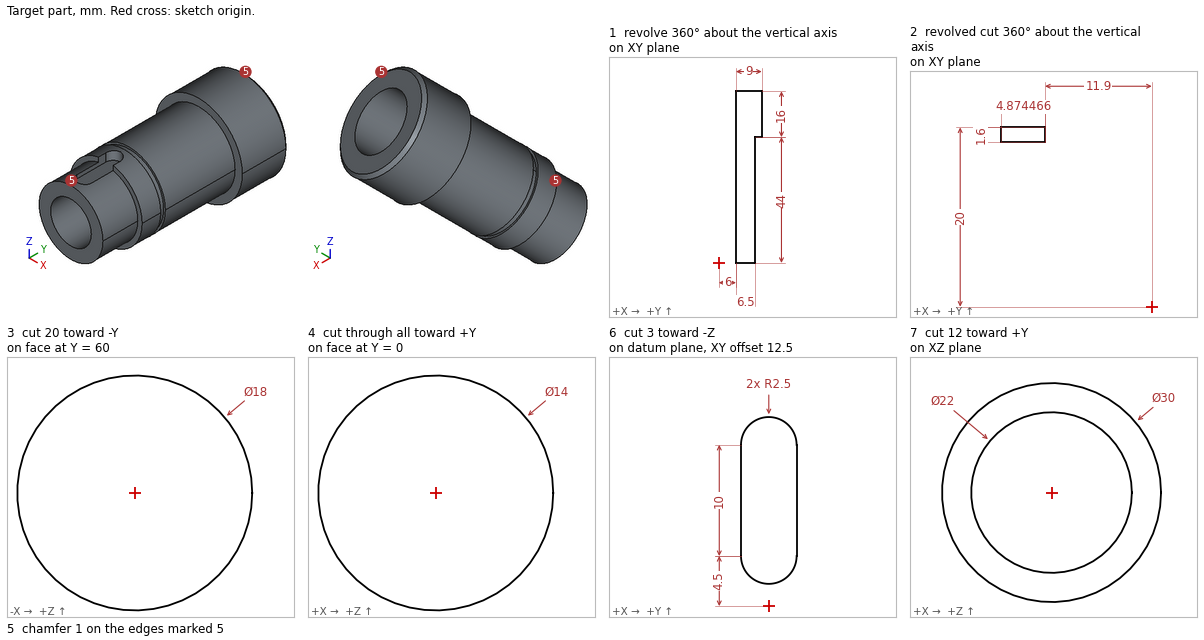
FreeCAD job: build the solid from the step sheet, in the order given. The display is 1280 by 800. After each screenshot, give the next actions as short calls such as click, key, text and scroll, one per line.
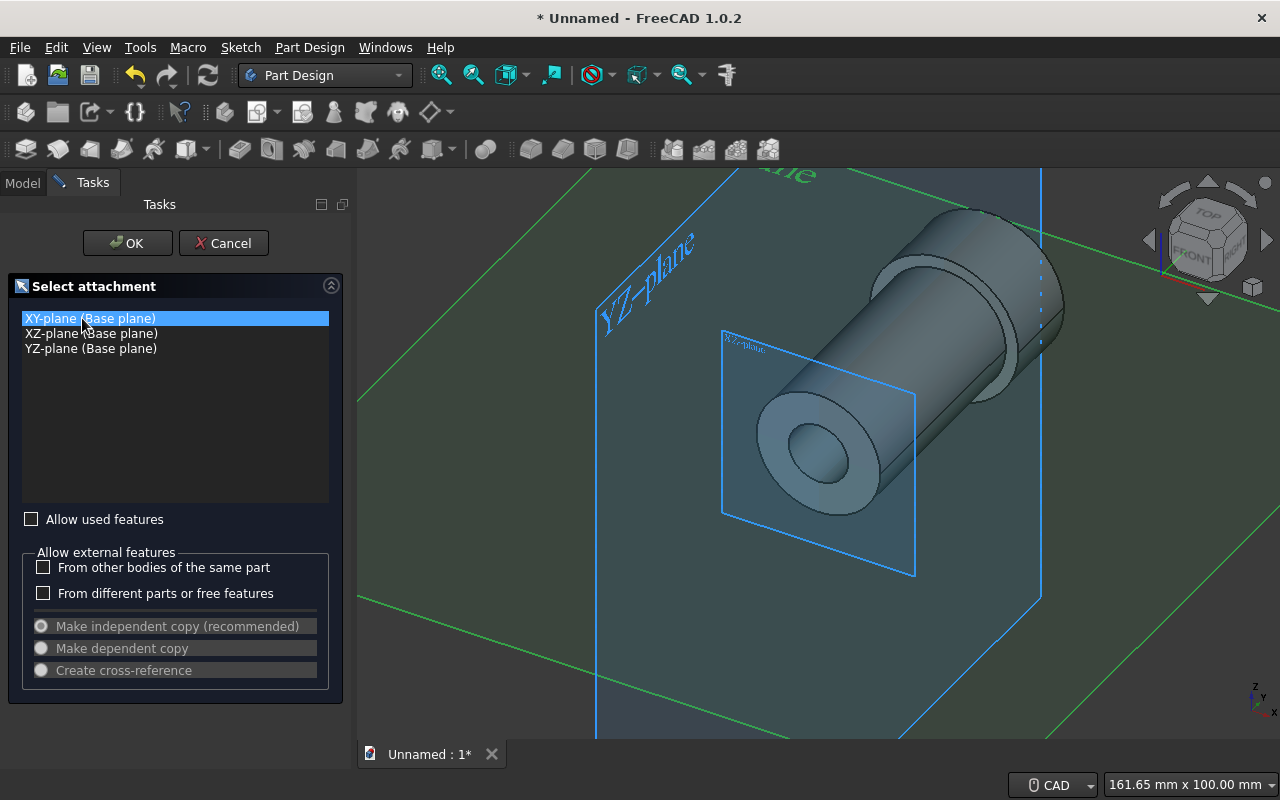
click(128, 243)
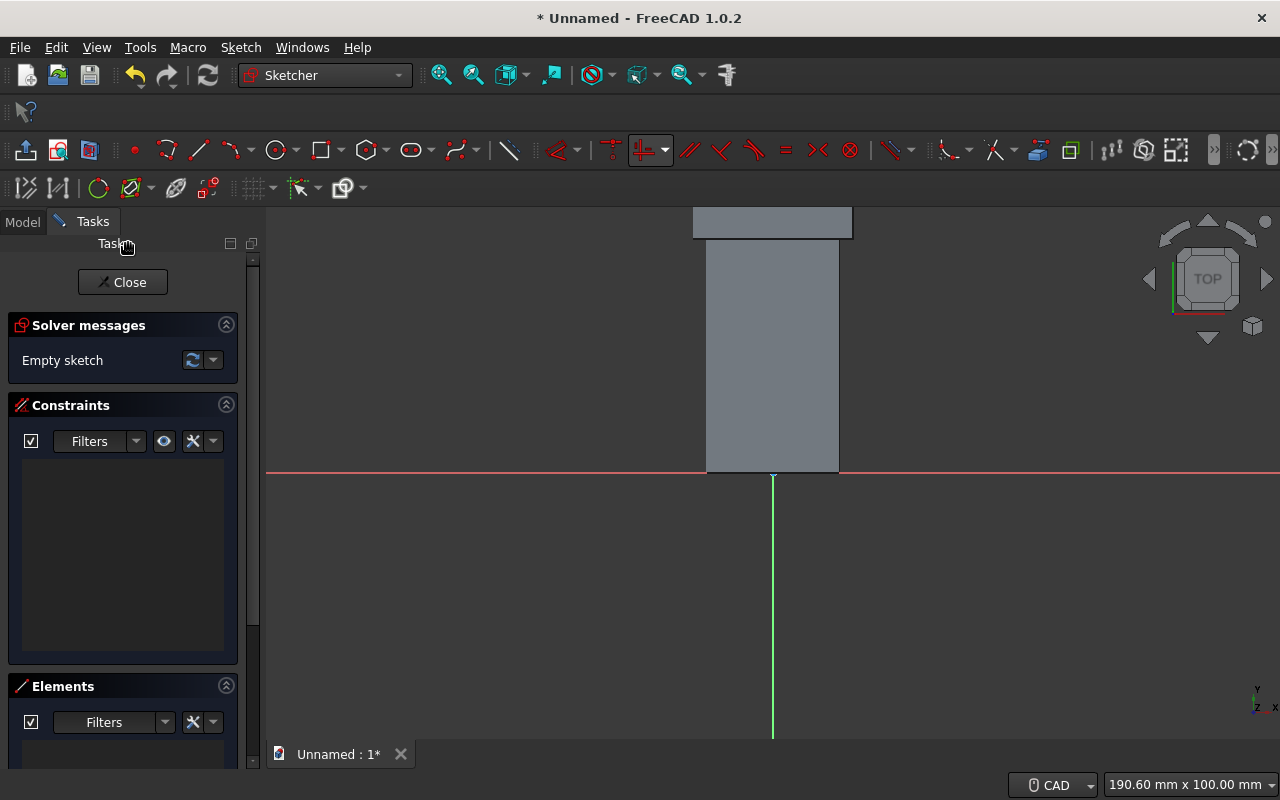
click(90, 150)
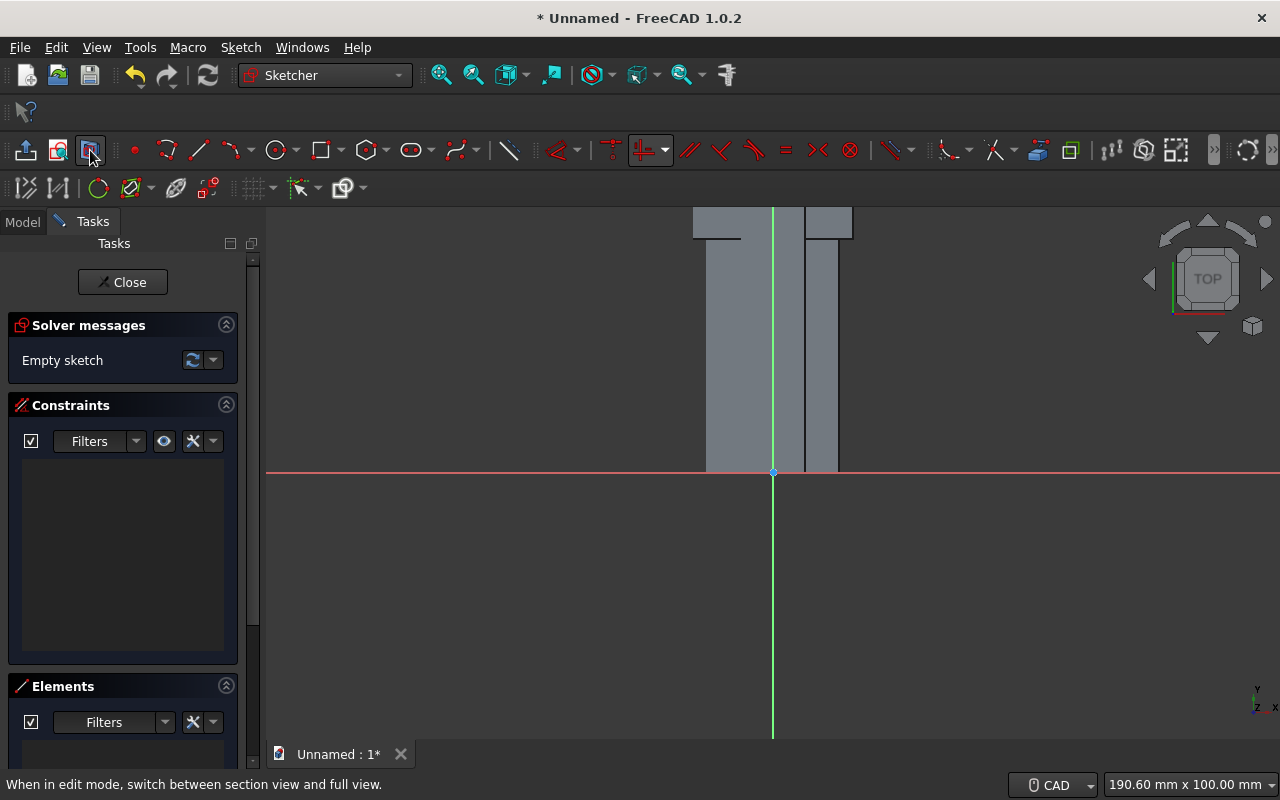
scroll(696, 366, up, 15)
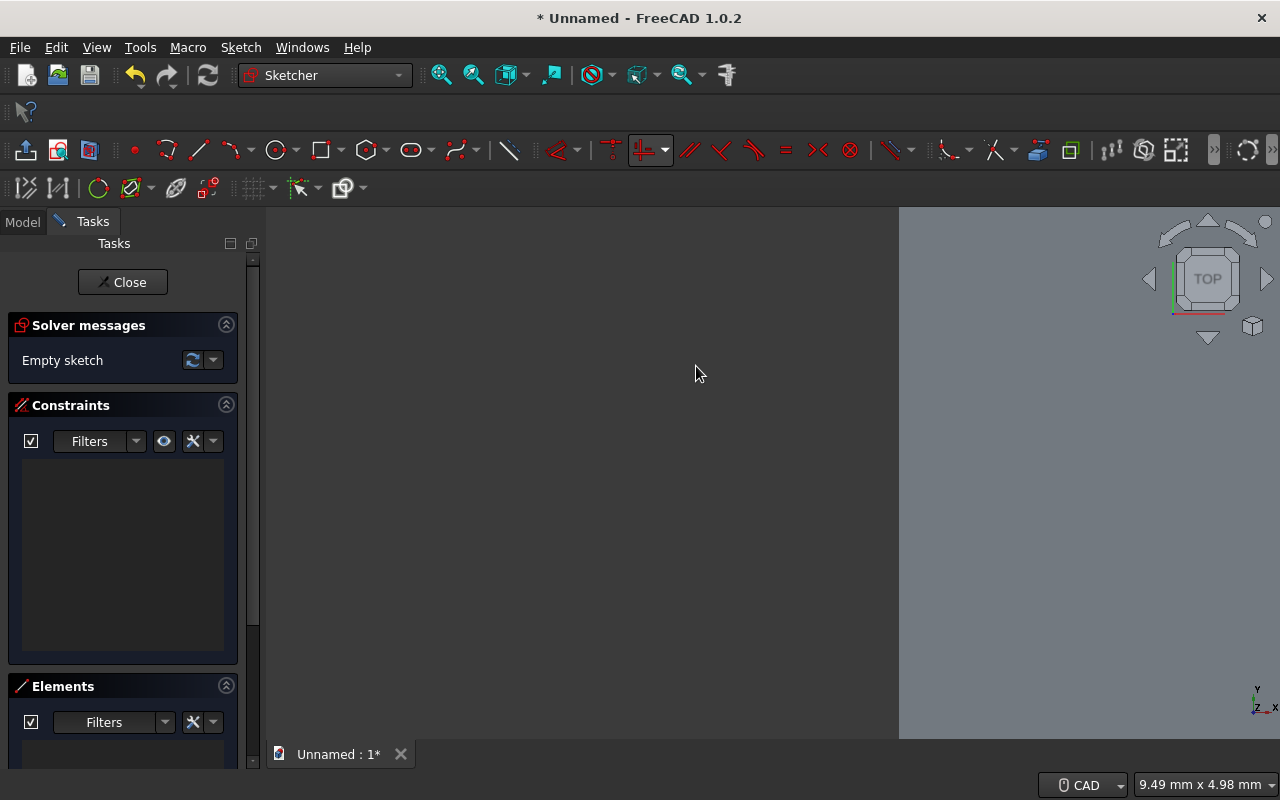
click(322, 150)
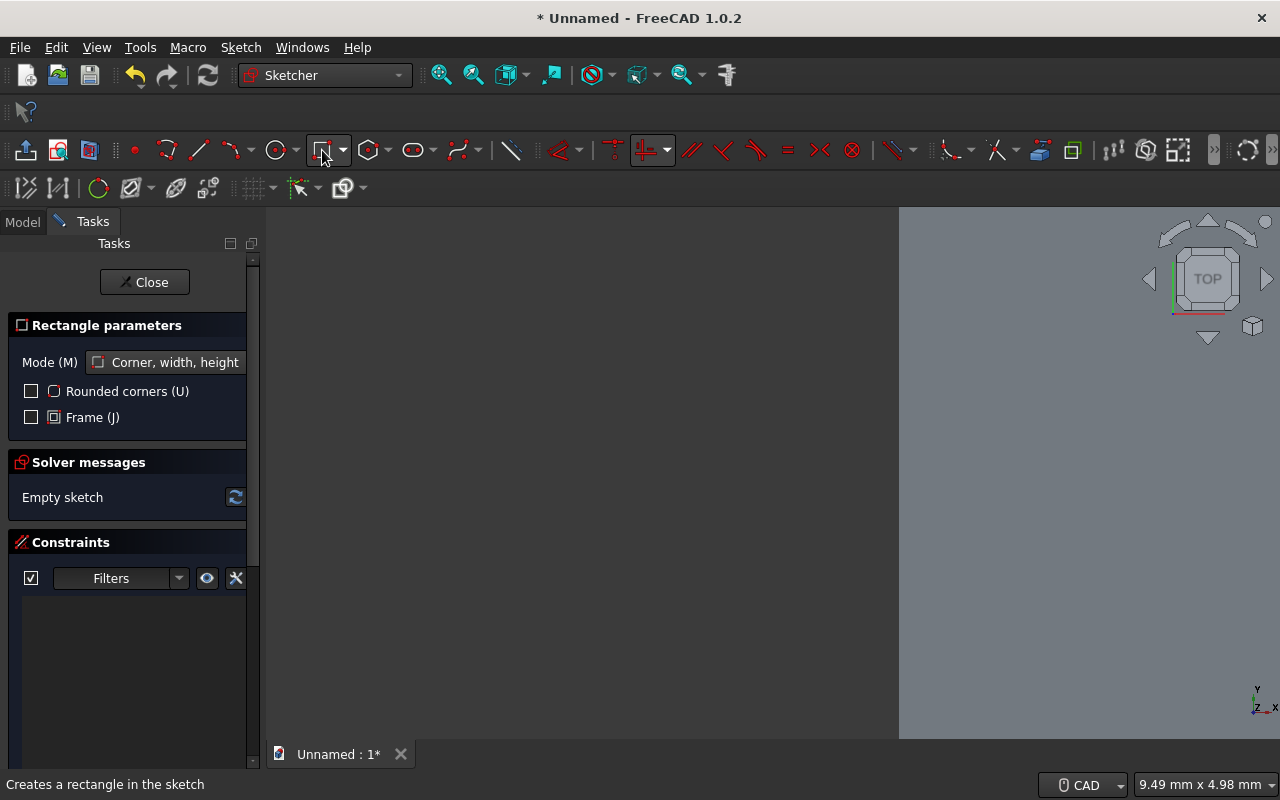
click(442, 372)
move(963, 543)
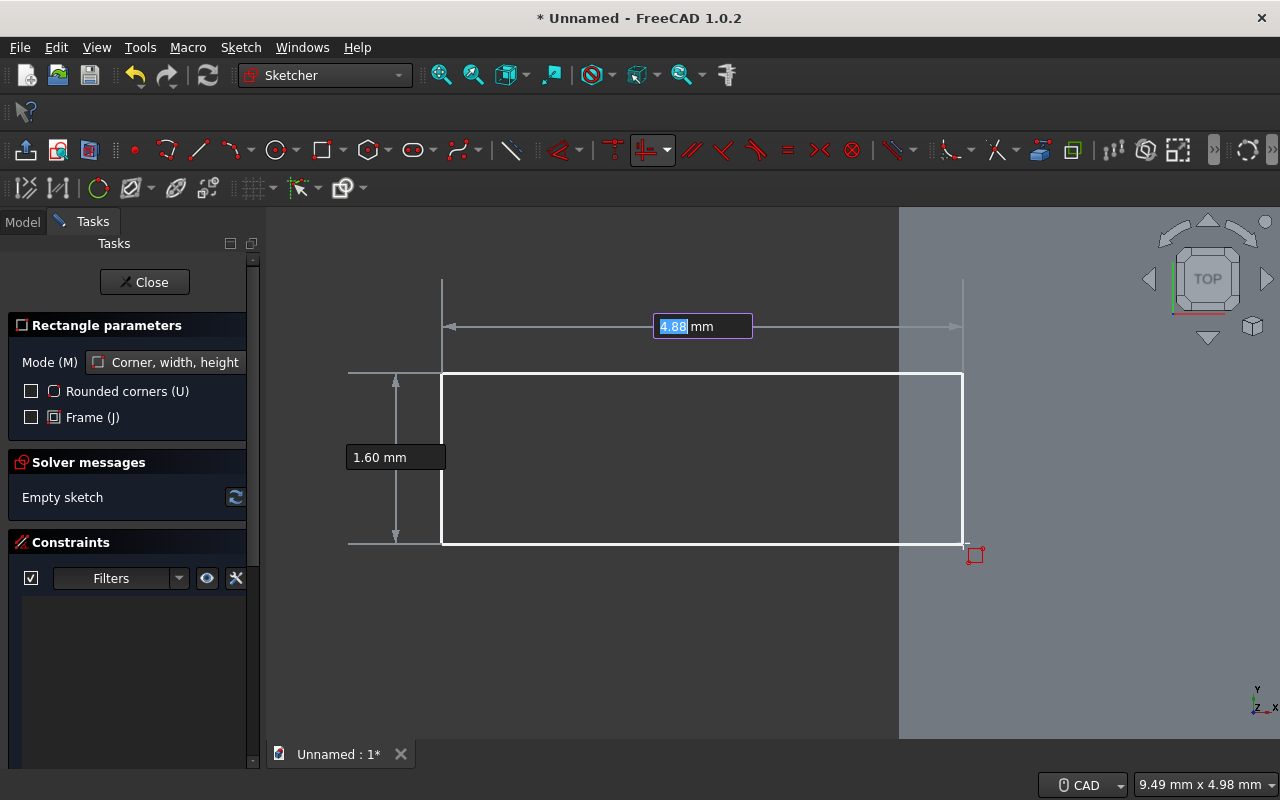
text(4.874466)
key(Tab)
text(1.6)
key(Return)
key(Escape)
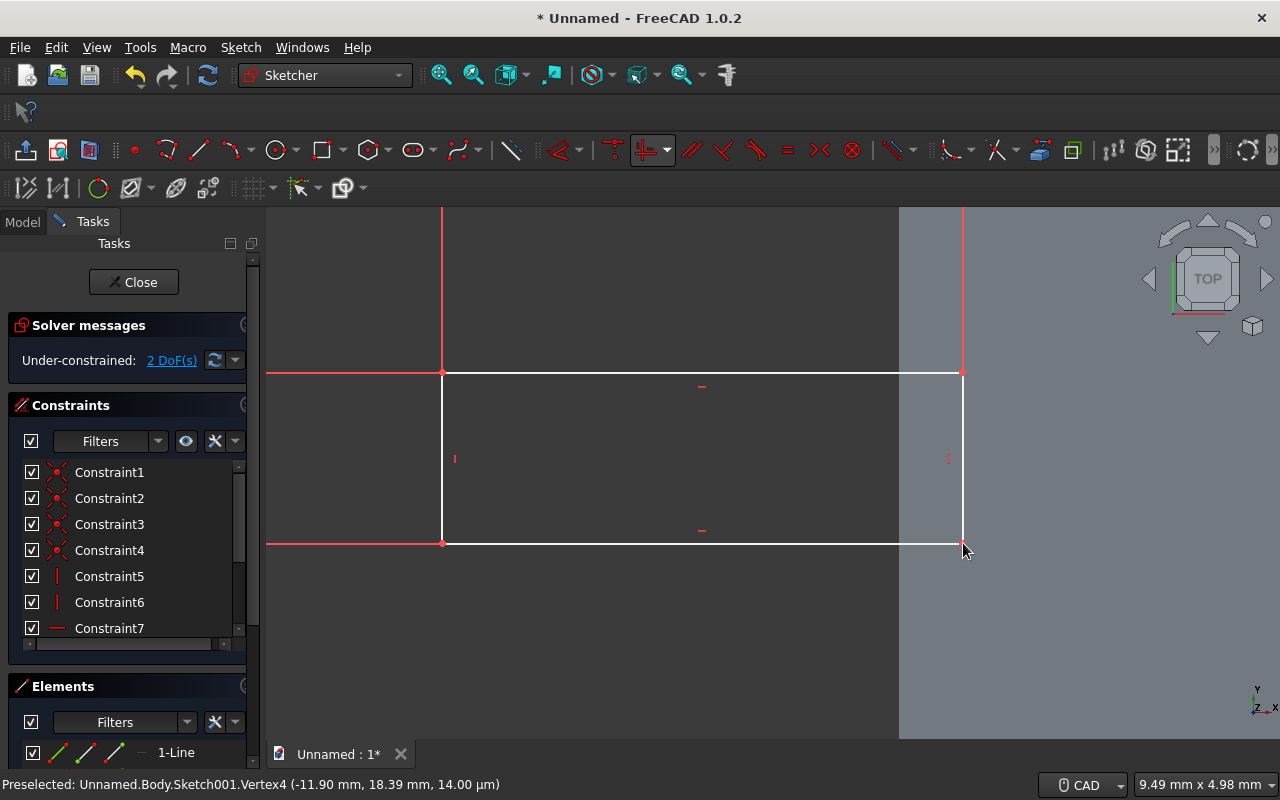
click(558, 150)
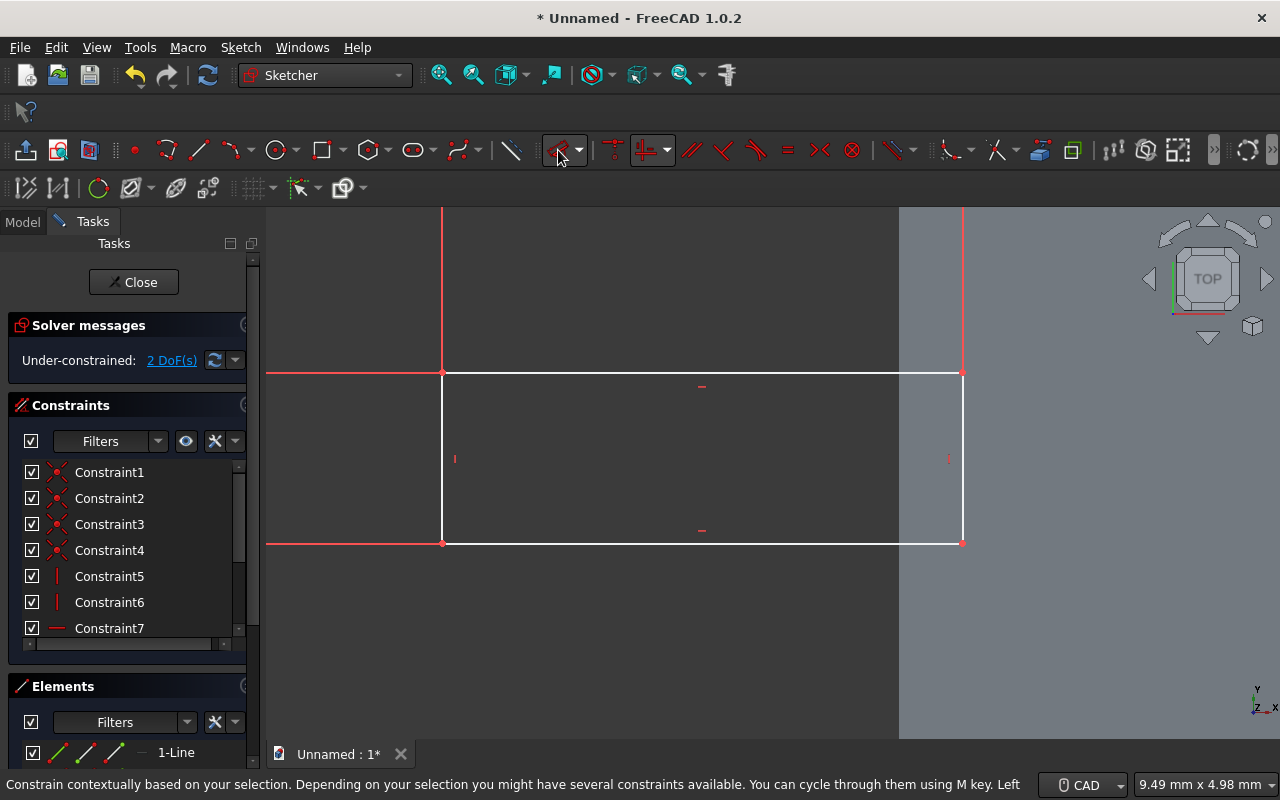
click(442, 373)
click(408, 542)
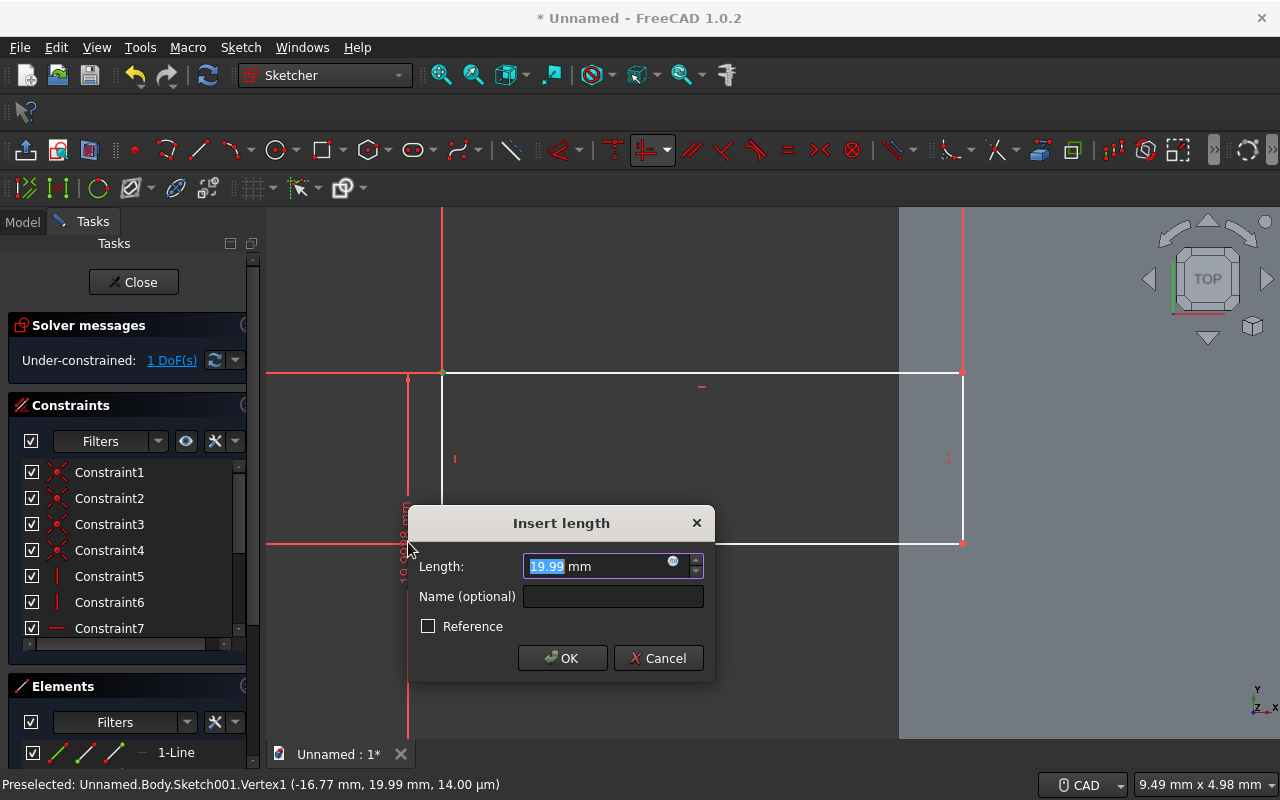
text(20)
key(Return)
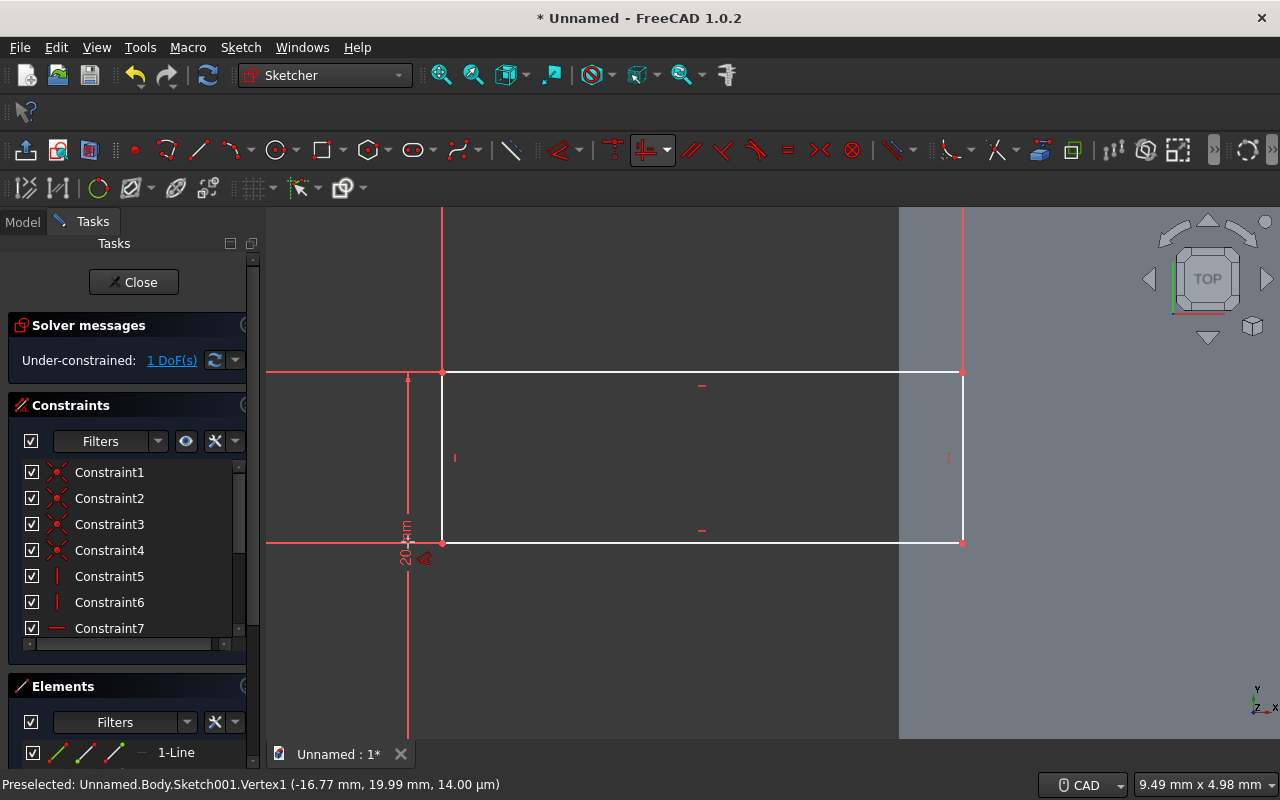
click(963, 543)
click(1039, 509)